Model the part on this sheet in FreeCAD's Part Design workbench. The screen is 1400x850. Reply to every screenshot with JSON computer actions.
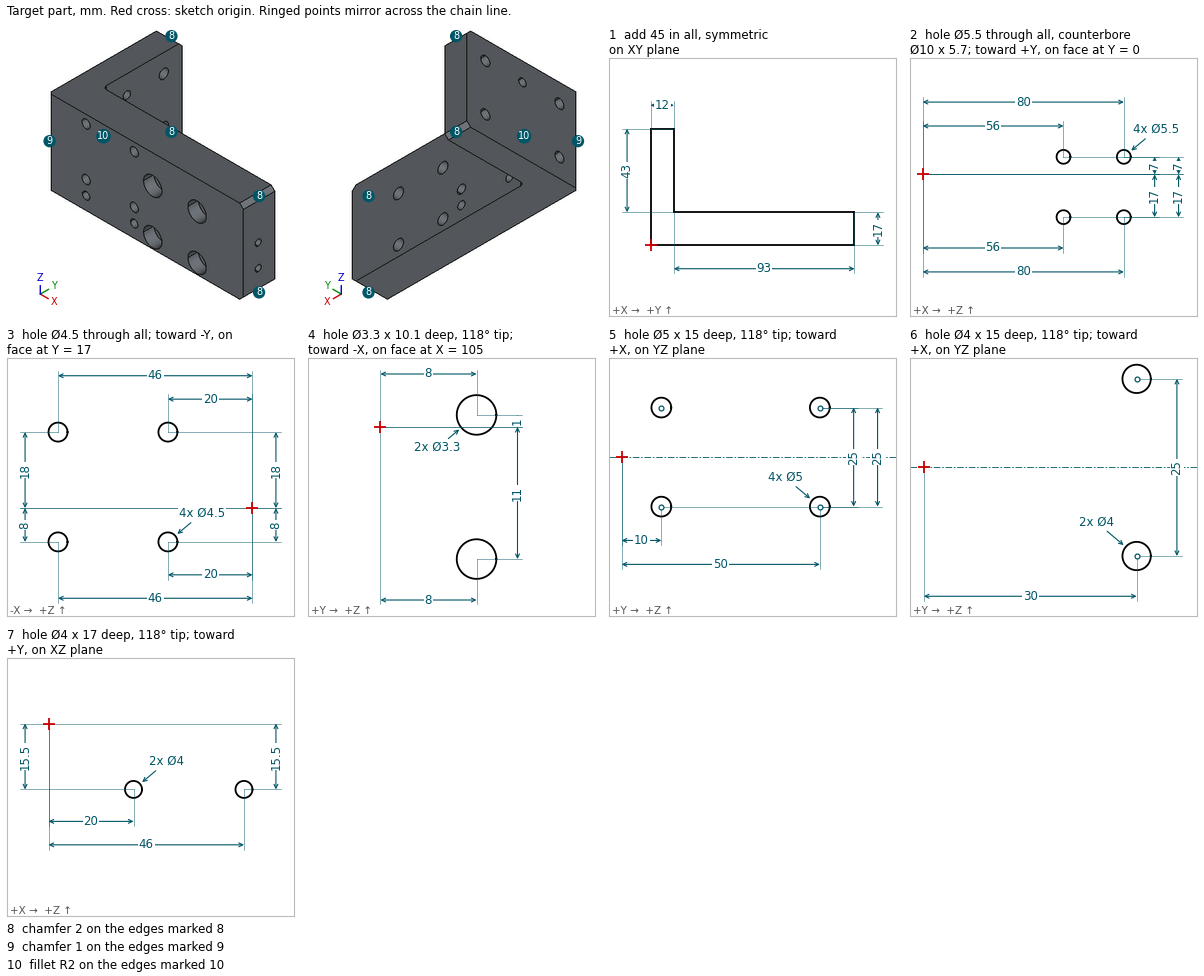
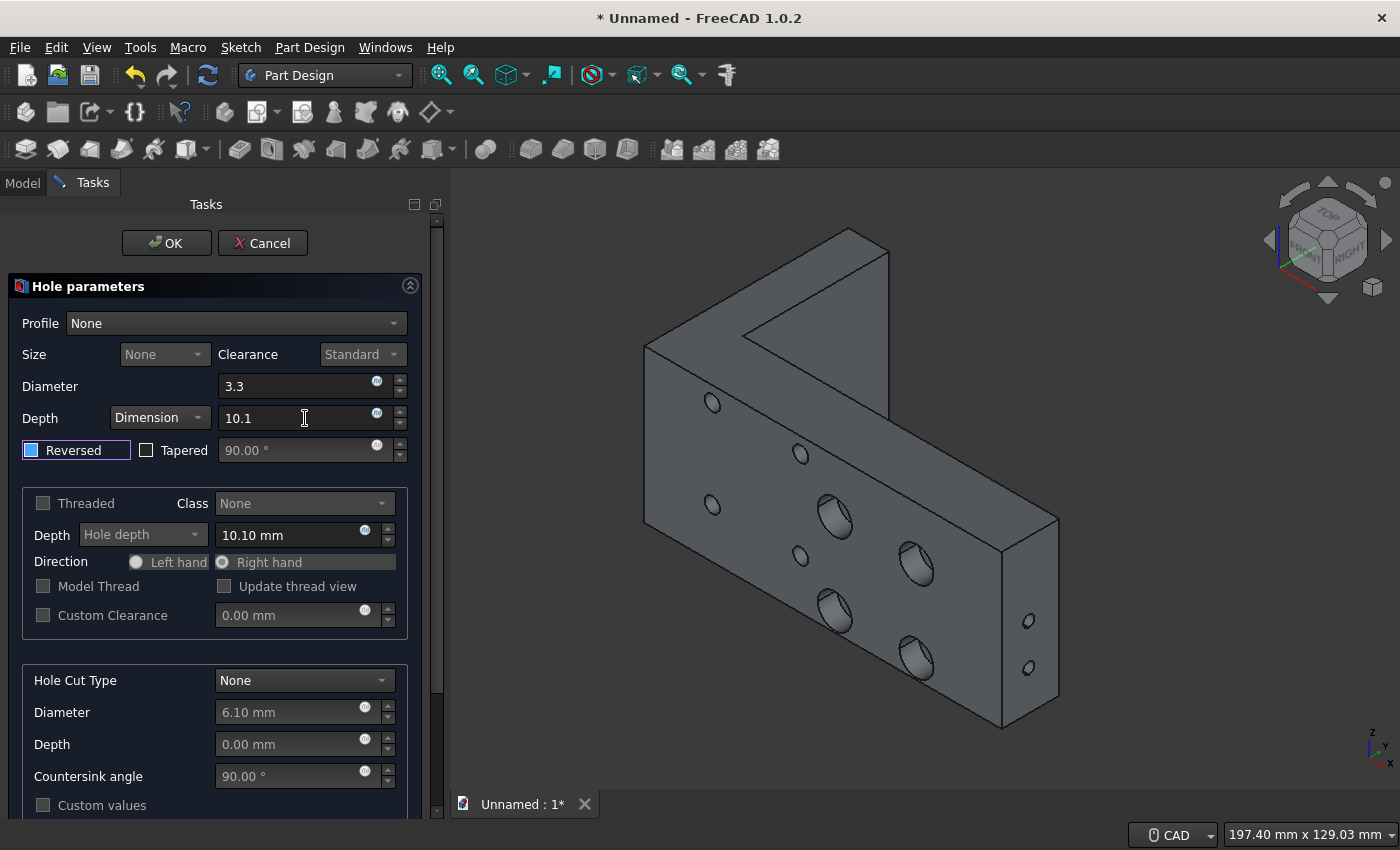
{"action": "left_click", "coordinate": [167, 243]}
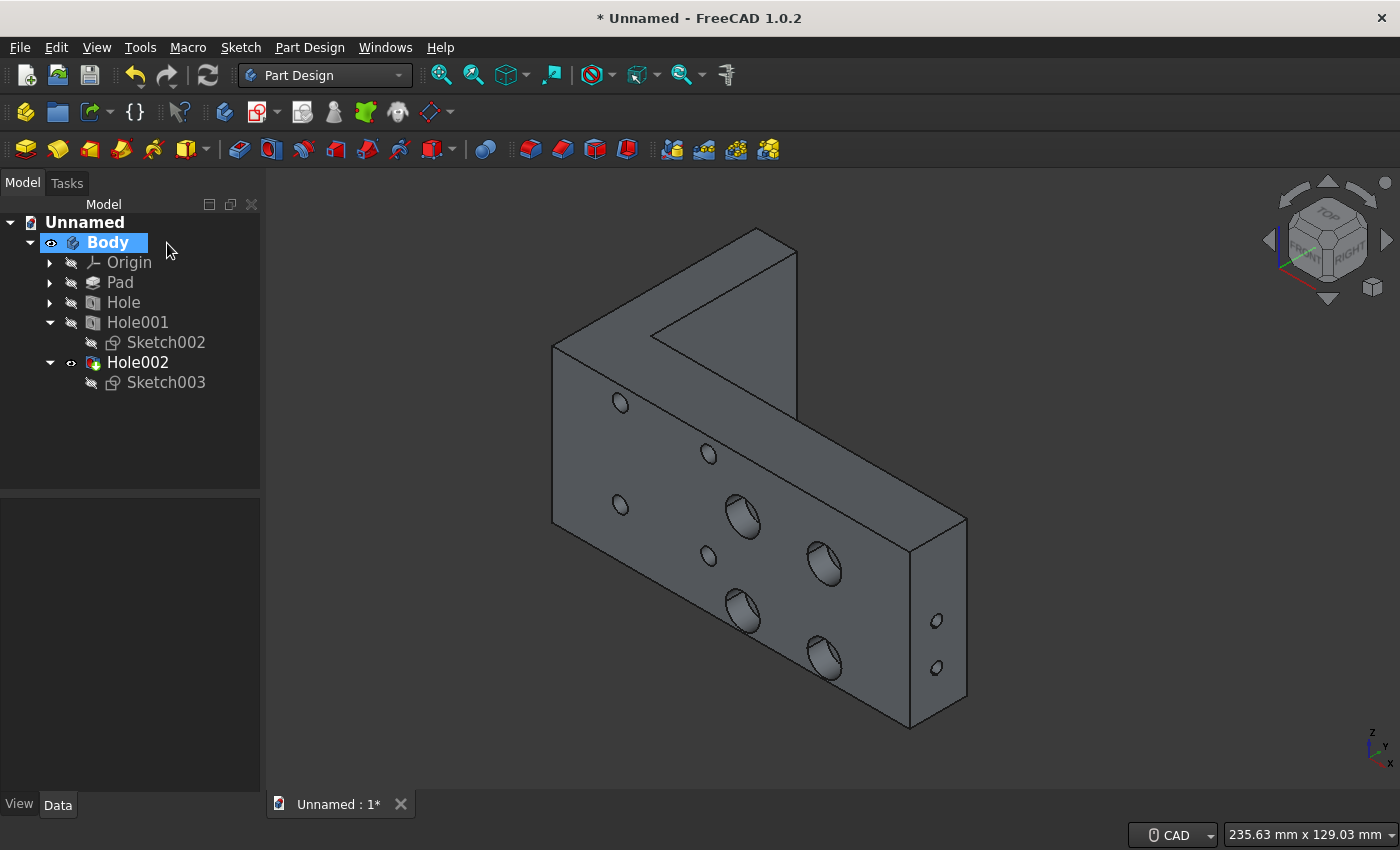
{"action": "left_click", "coordinate": [258, 112]}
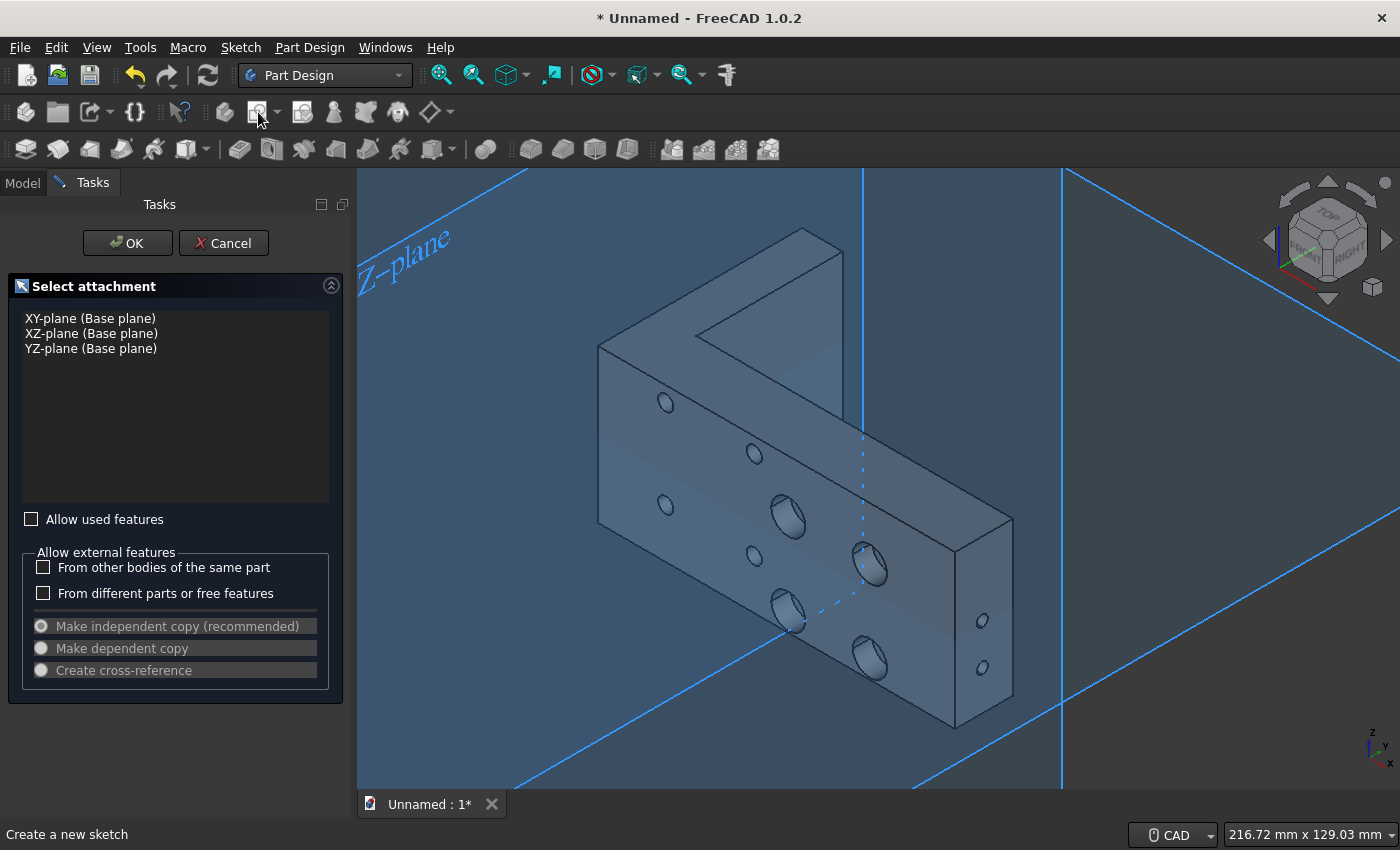
{"action": "left_click", "coordinate": [82, 348]}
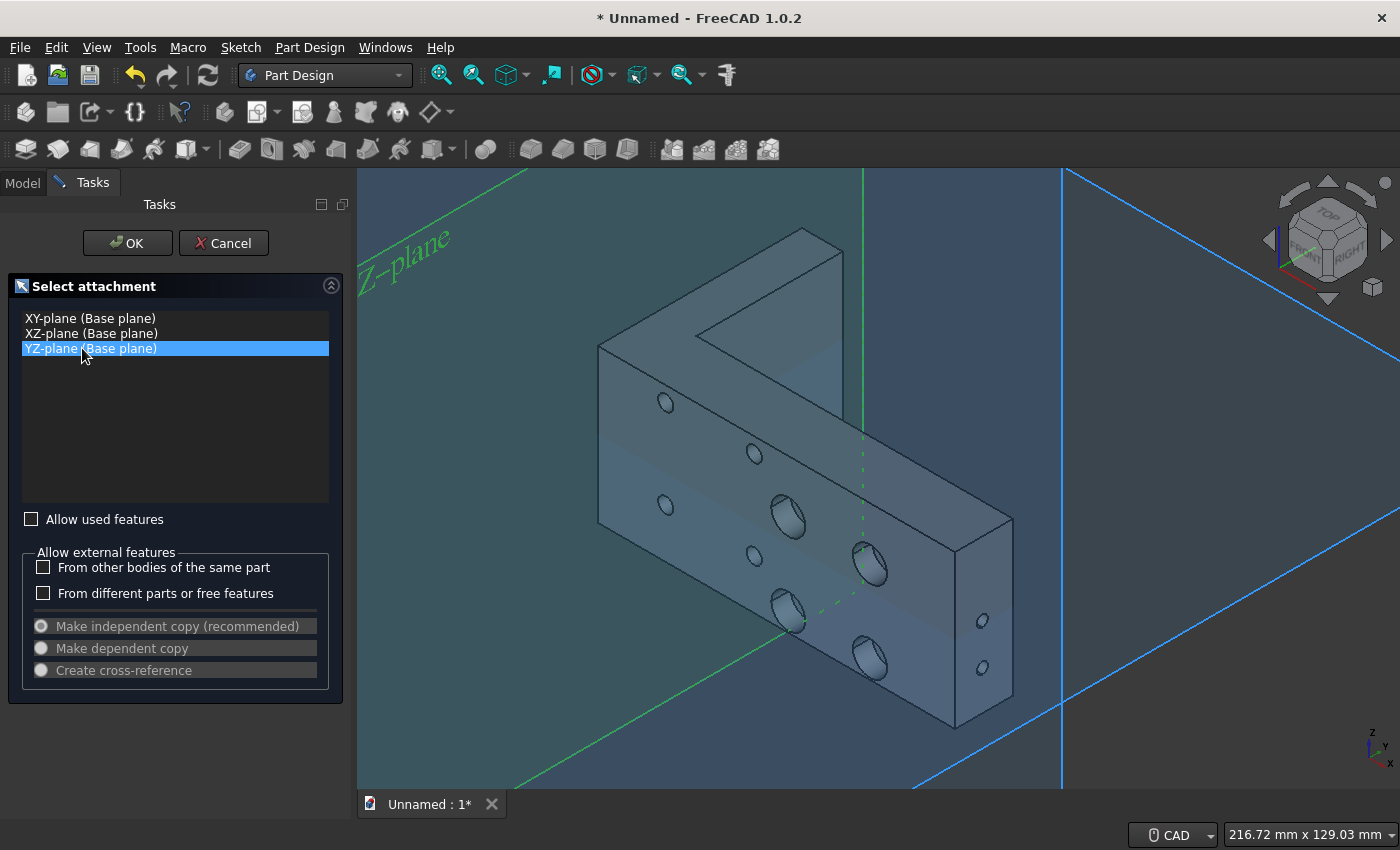
{"action": "left_click", "coordinate": [128, 243]}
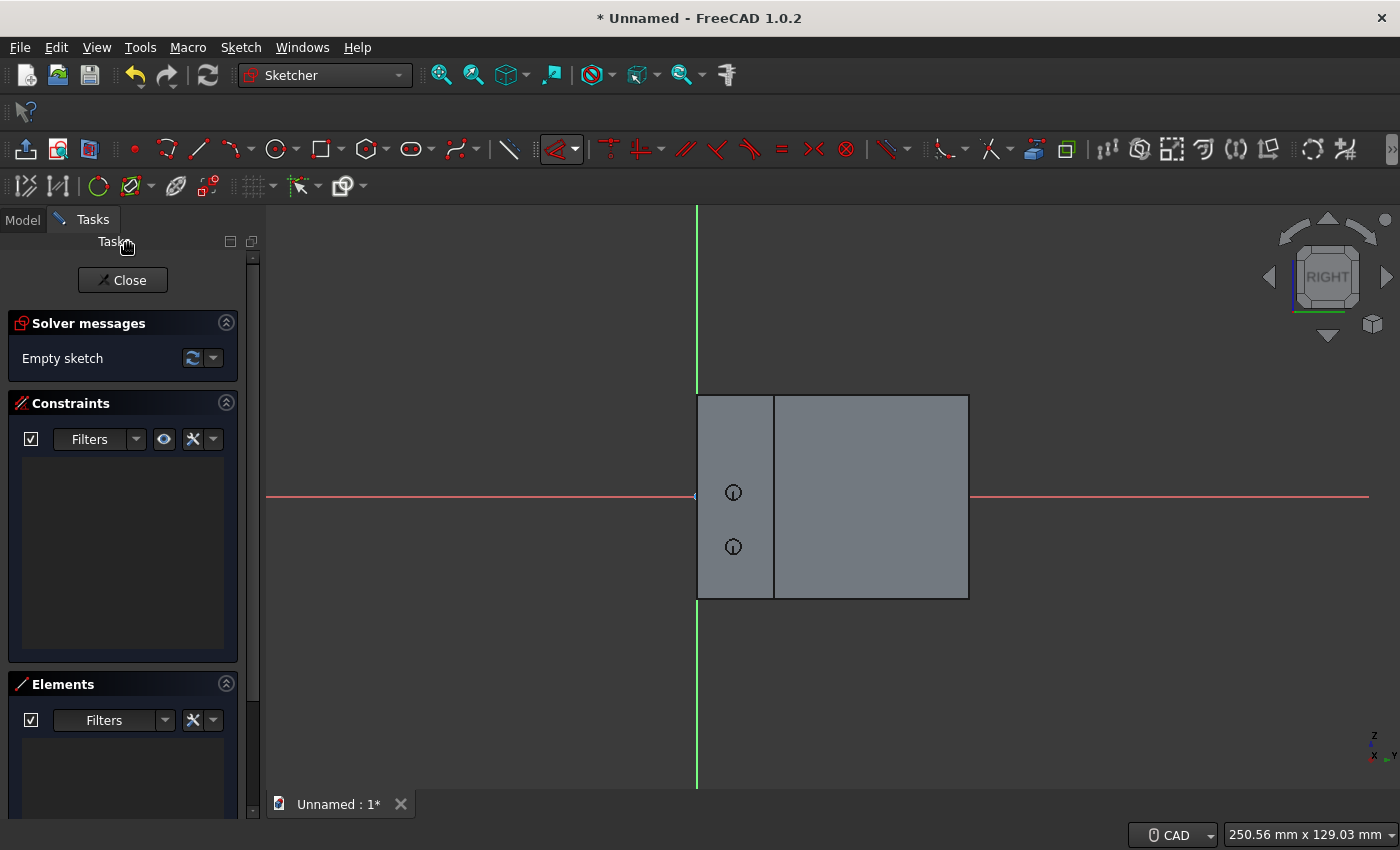
{"action": "key", "text": "q s"}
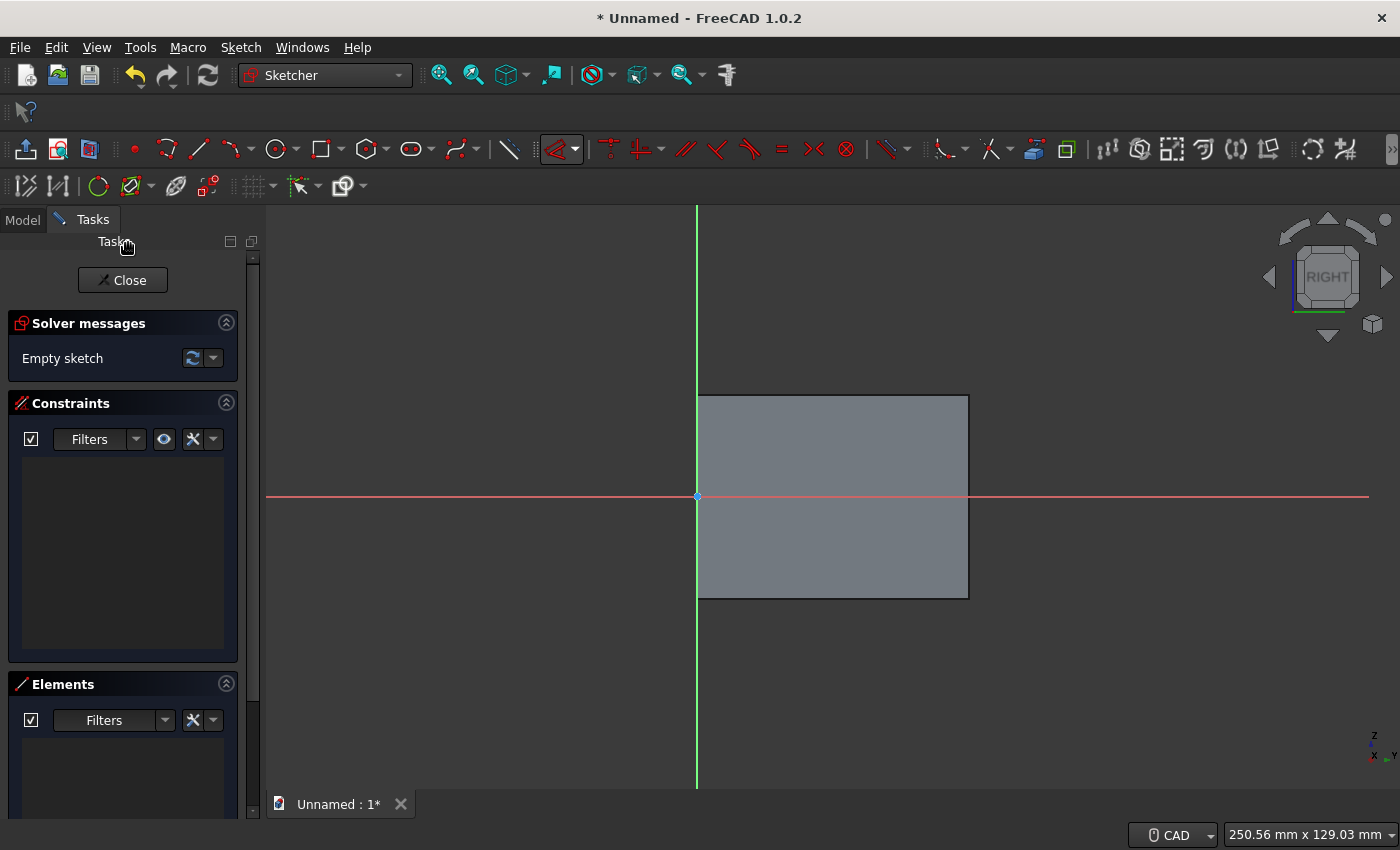
{"action": "scroll", "coordinate": [846, 497], "scroll_direction": "up", "scroll_amount": 5}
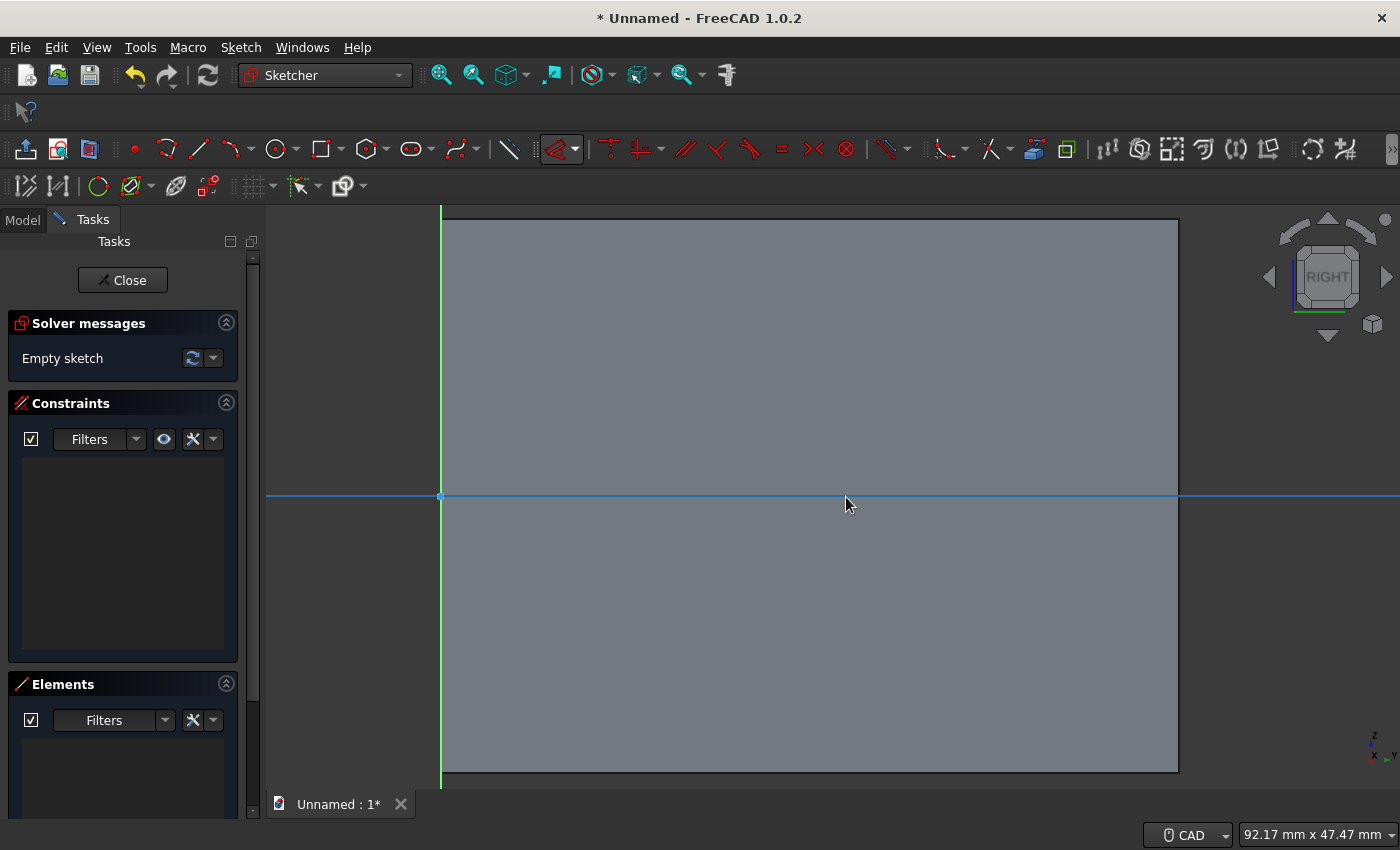
{"action": "key", "text": "g c"}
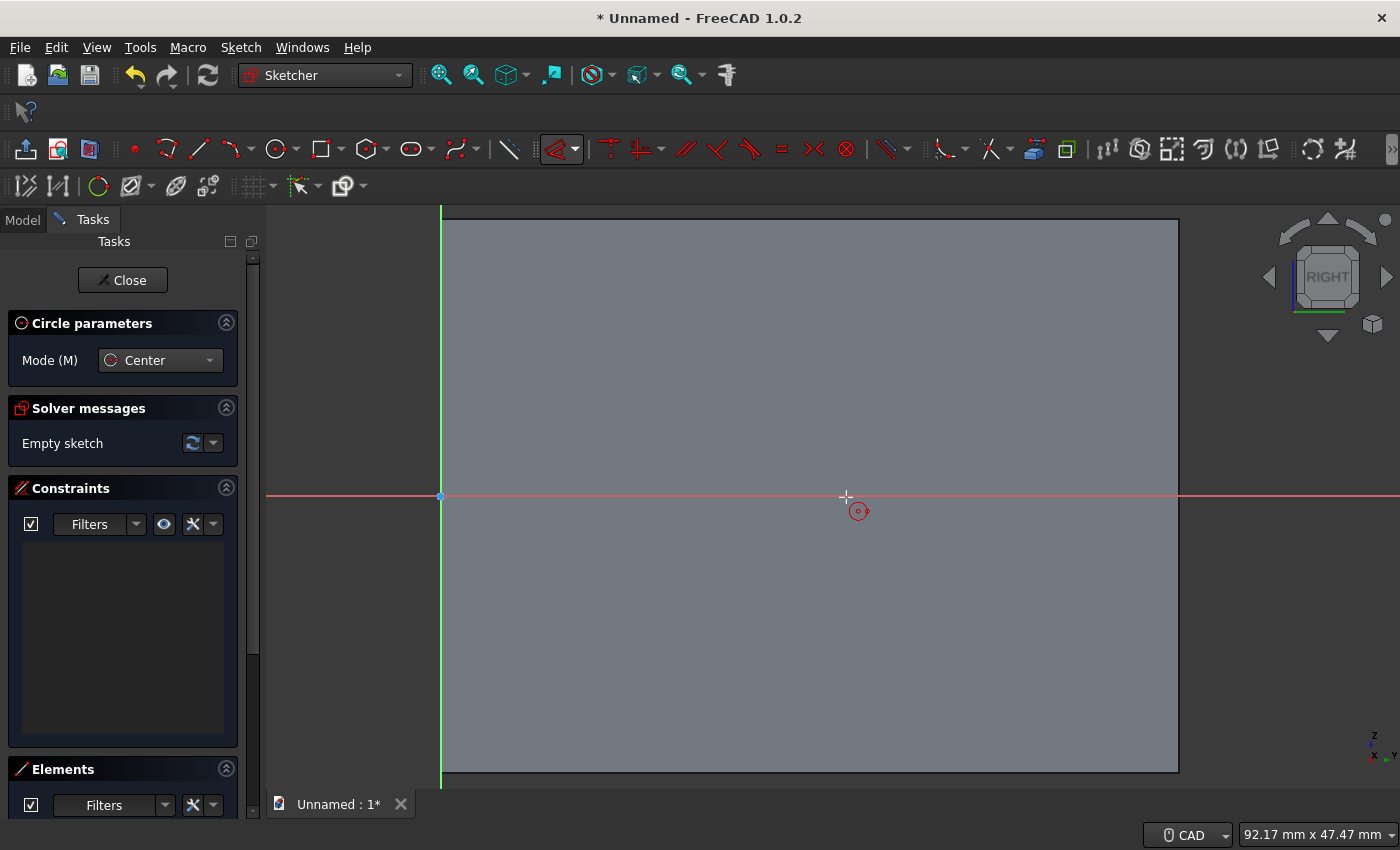
{"action": "left_click", "coordinate": [1056, 650]}
{"action": "left_click", "coordinate": [1078, 628]}